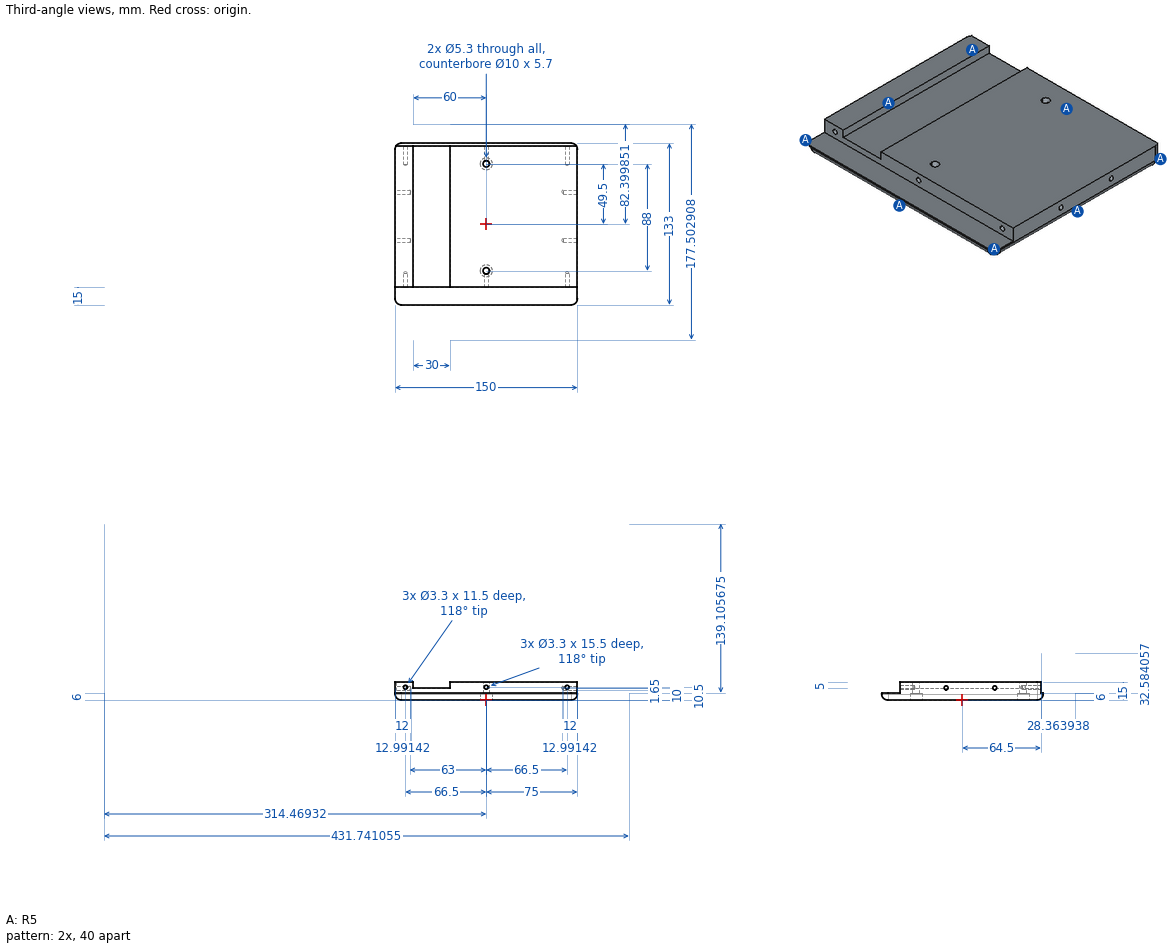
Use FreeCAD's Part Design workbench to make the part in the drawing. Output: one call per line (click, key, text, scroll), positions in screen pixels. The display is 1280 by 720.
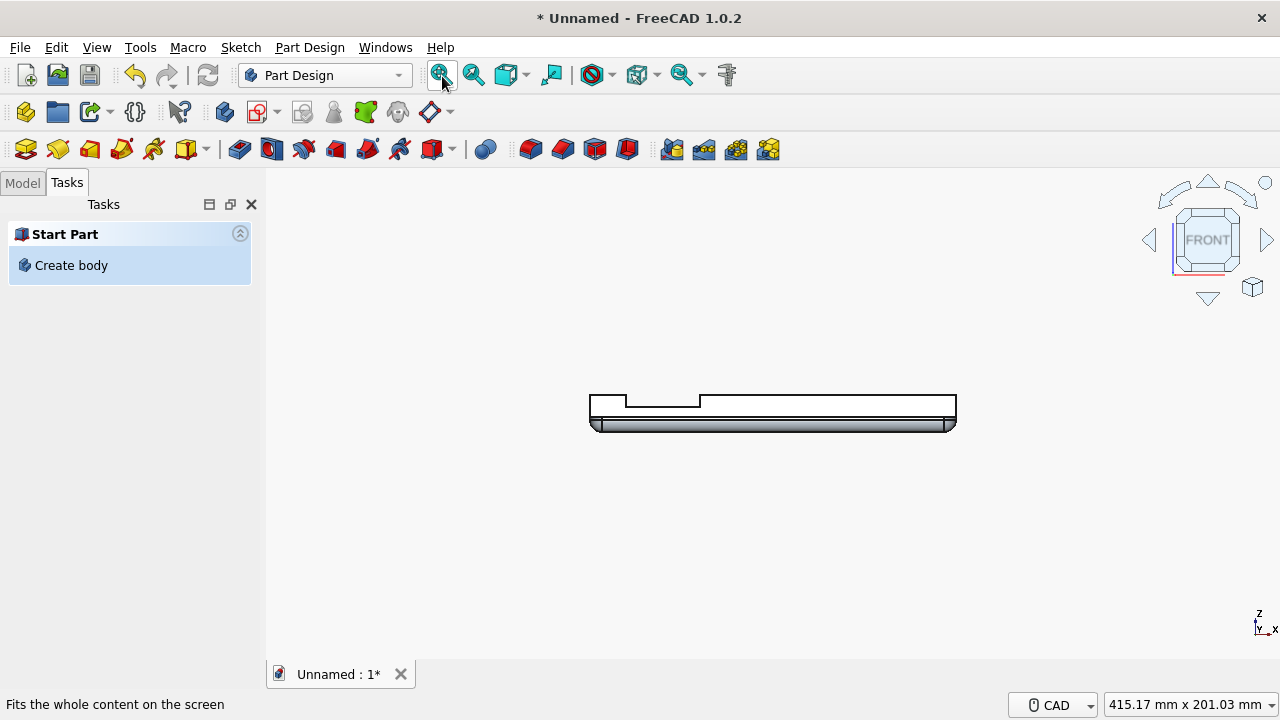
click(930, 405)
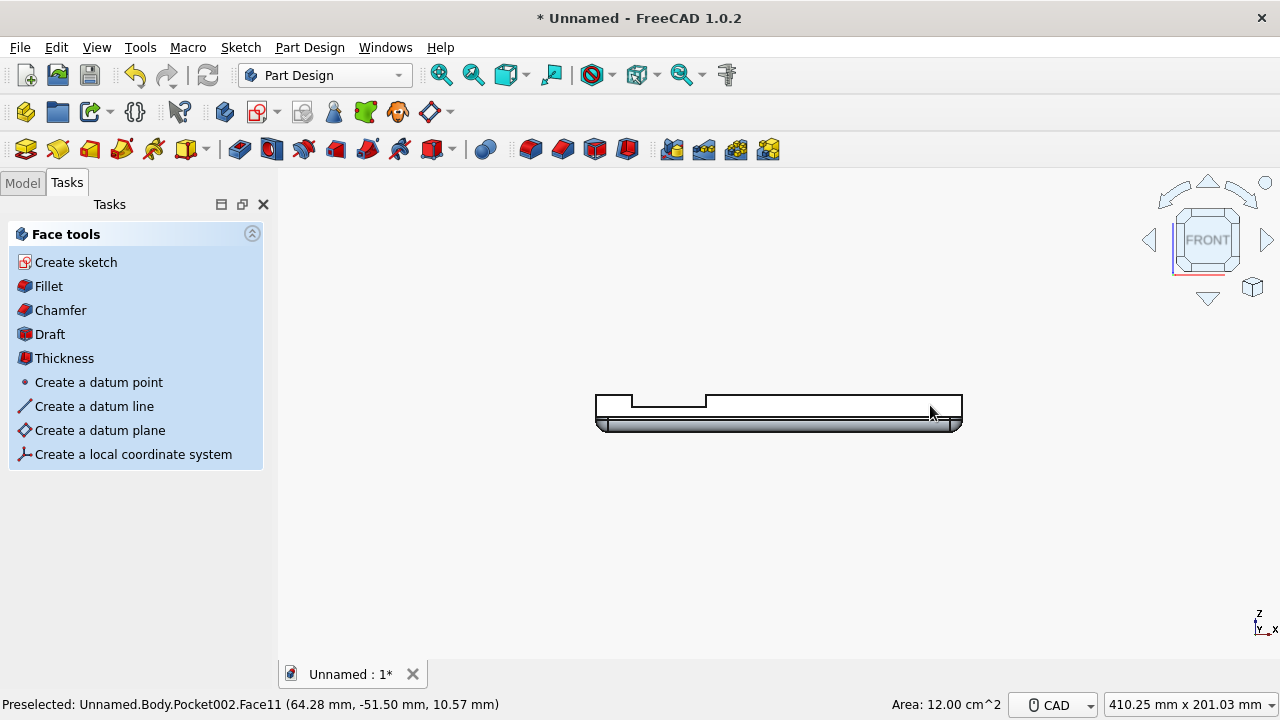
click(258, 112)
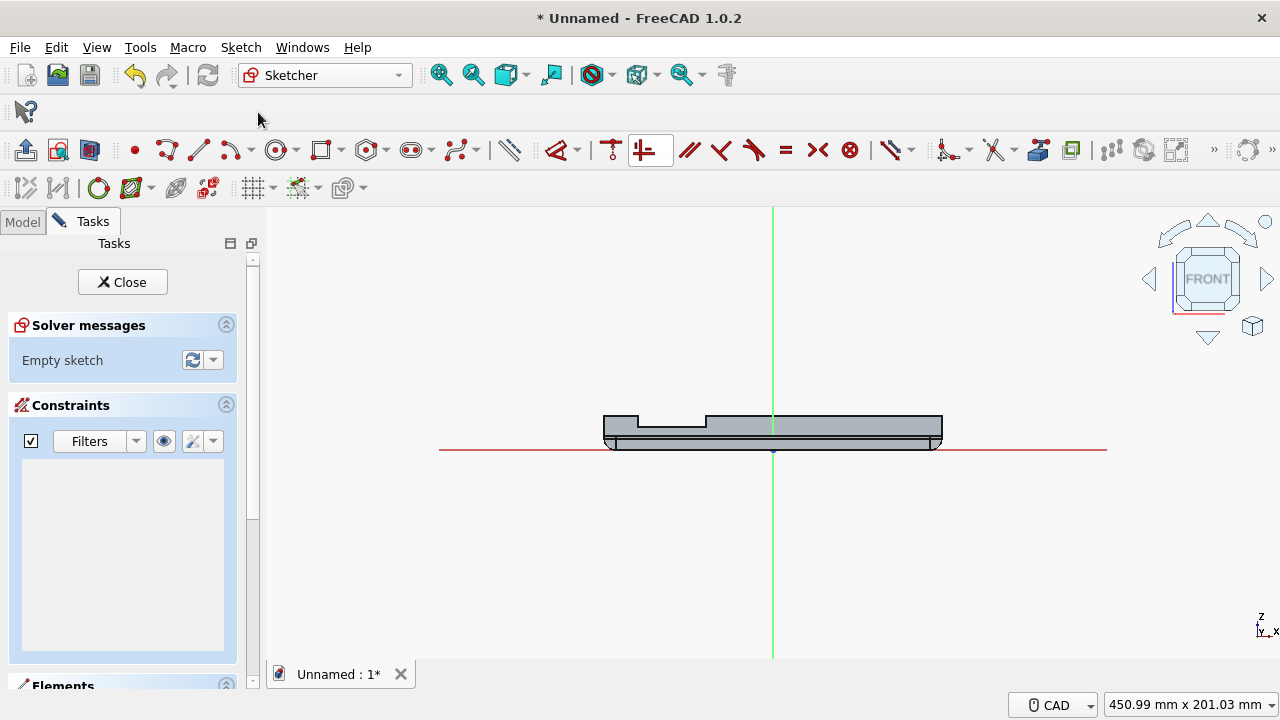
click(90, 150)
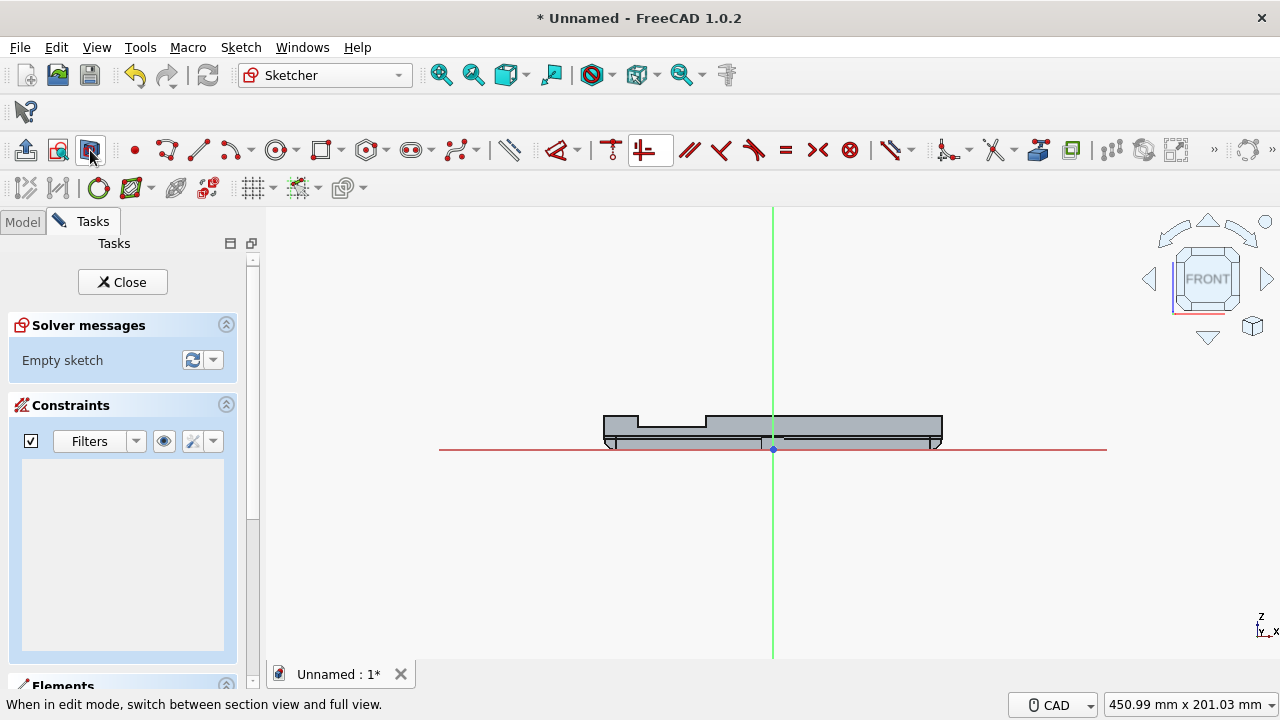
scroll(856, 440, up, 3)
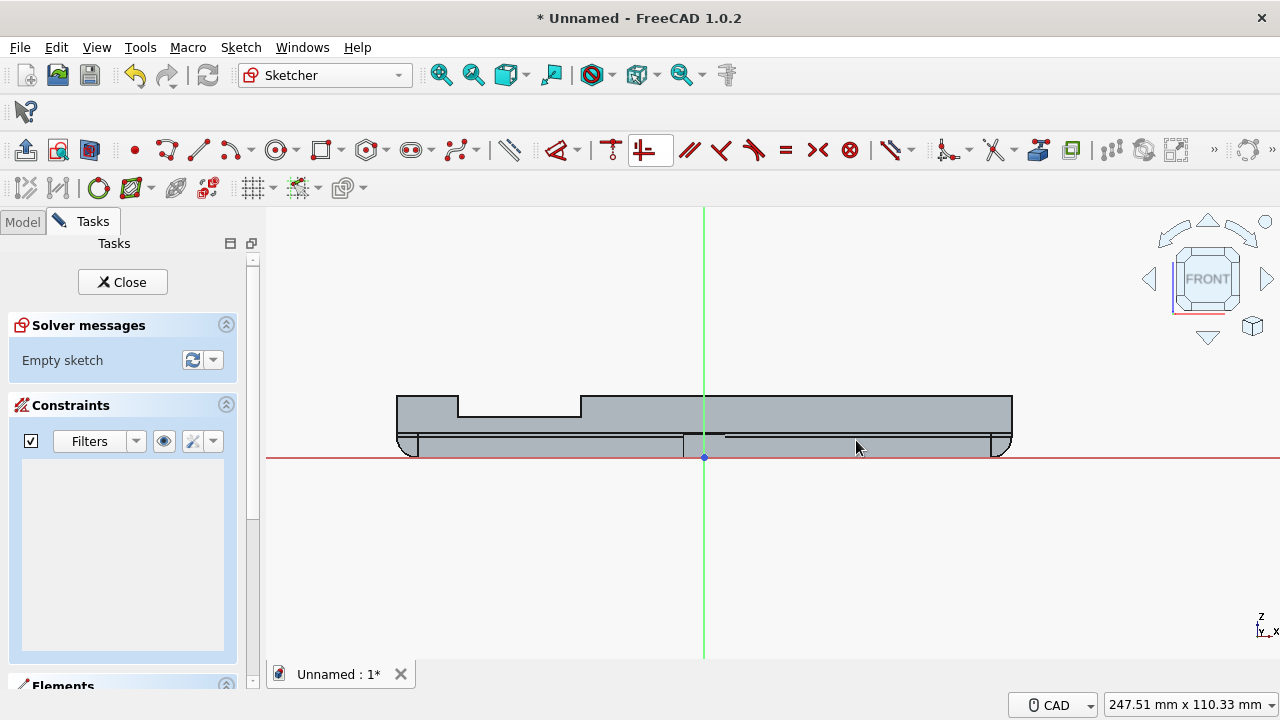
click(276, 150)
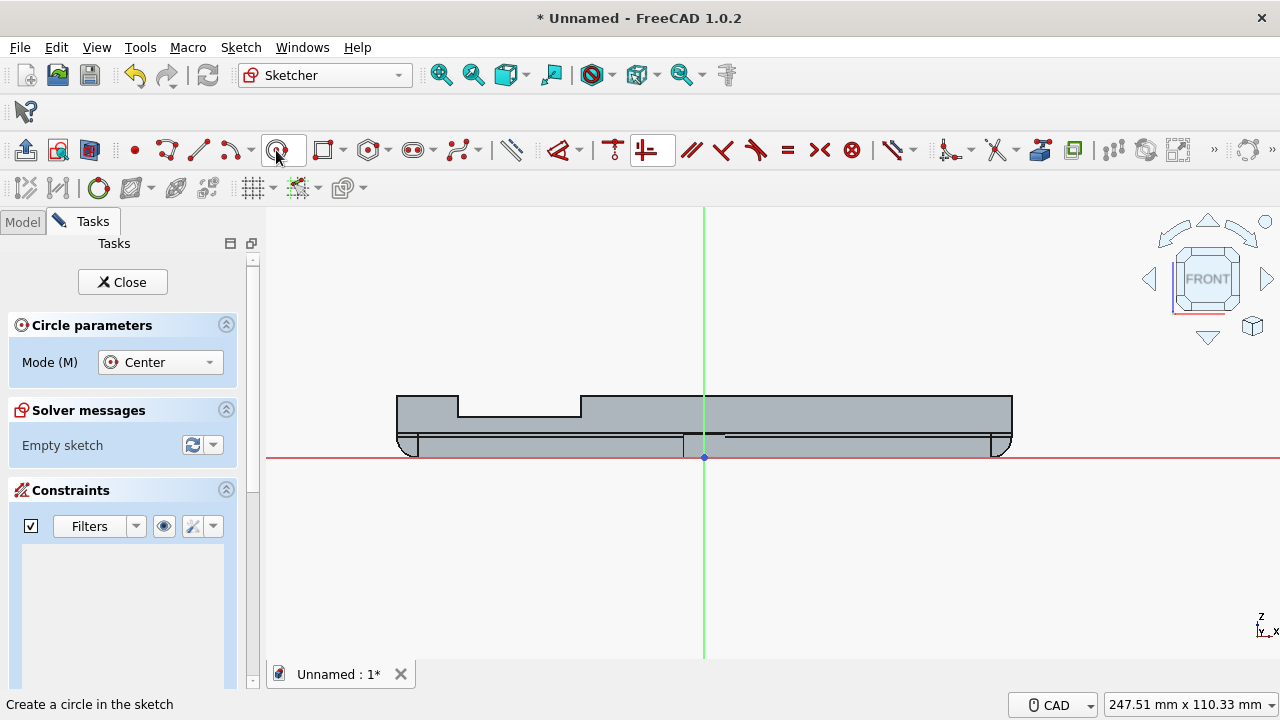
scroll(432, 415, up, 7)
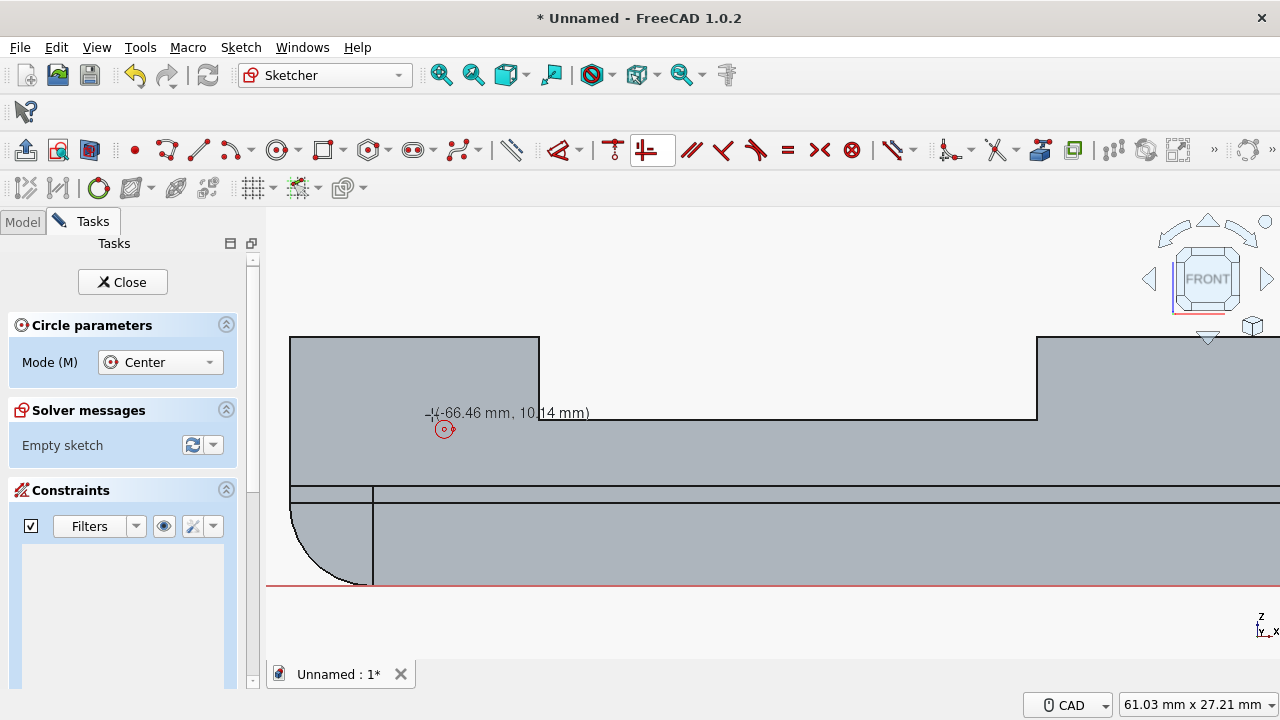
scroll(432, 416, down, 7)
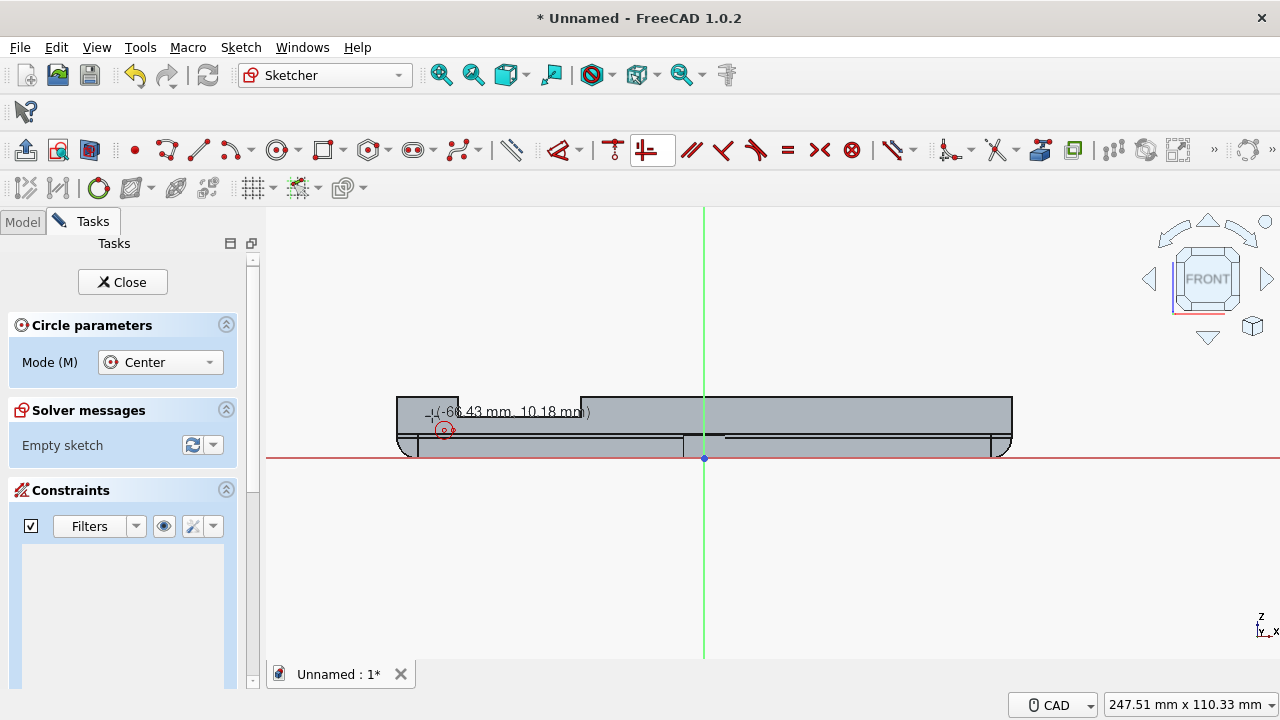
click(432, 415)
move(437, 411)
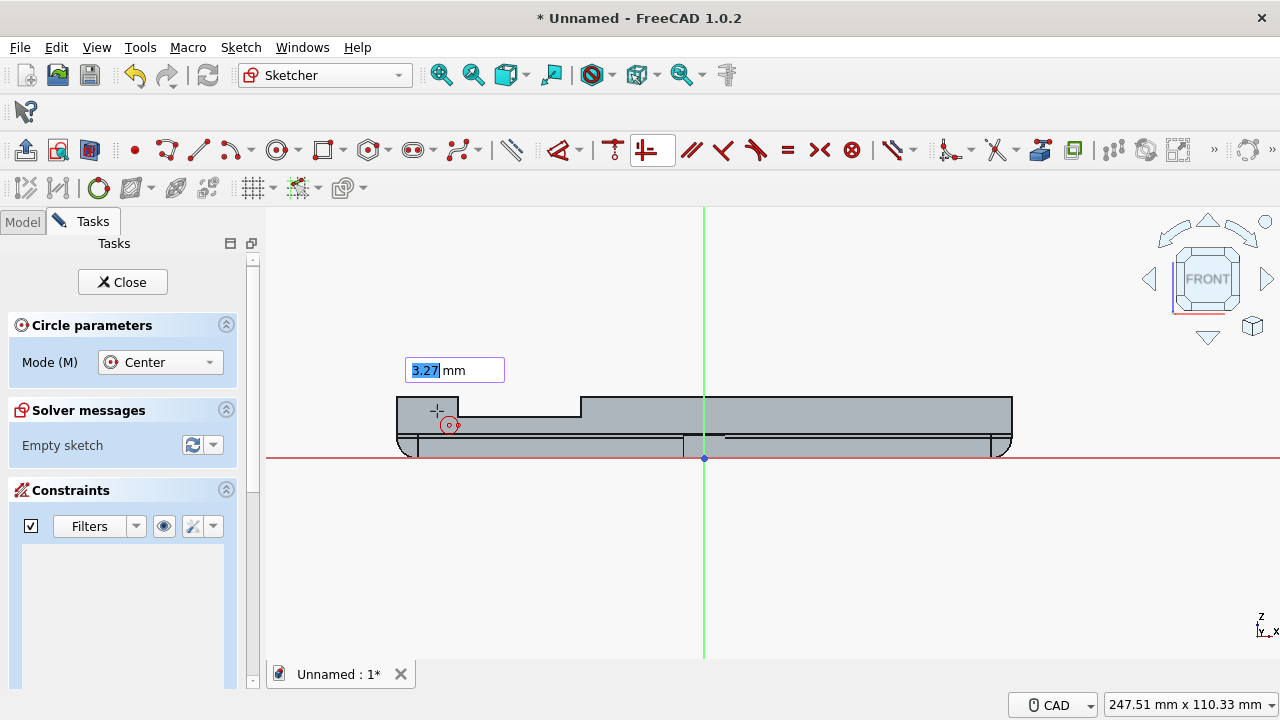
text(3.3)
key(Return)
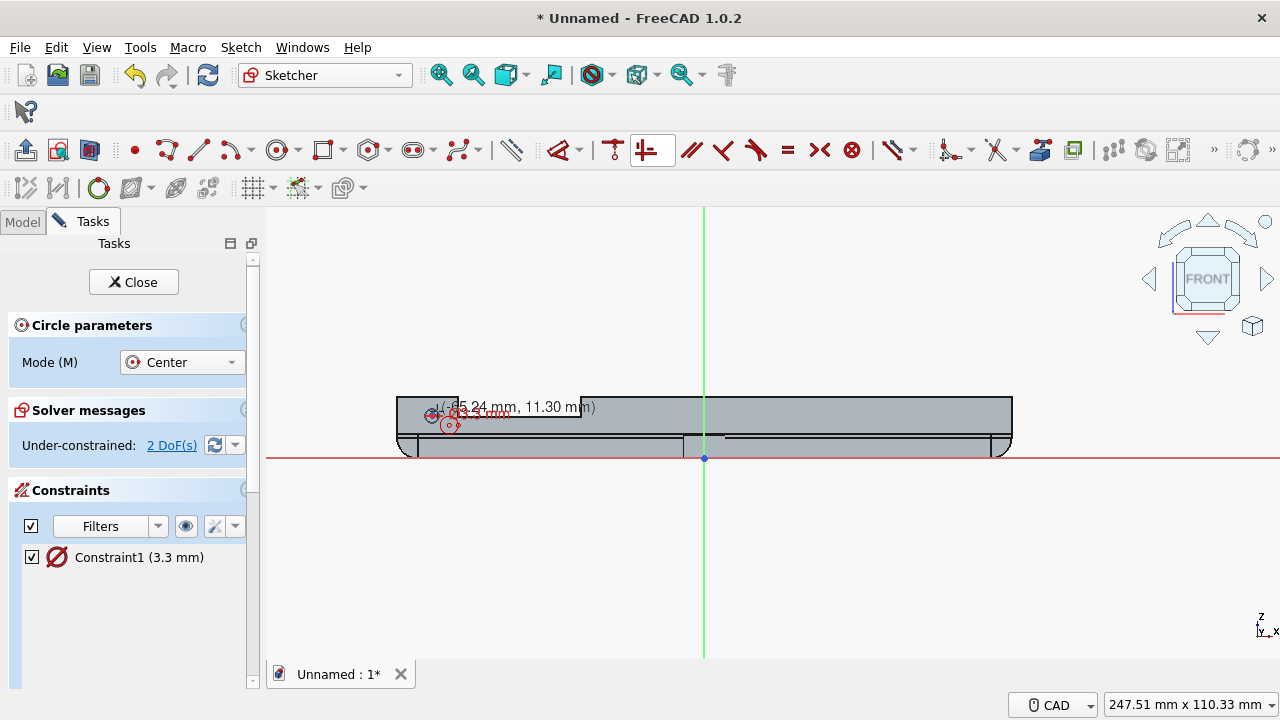
scroll(704, 415, up, 7)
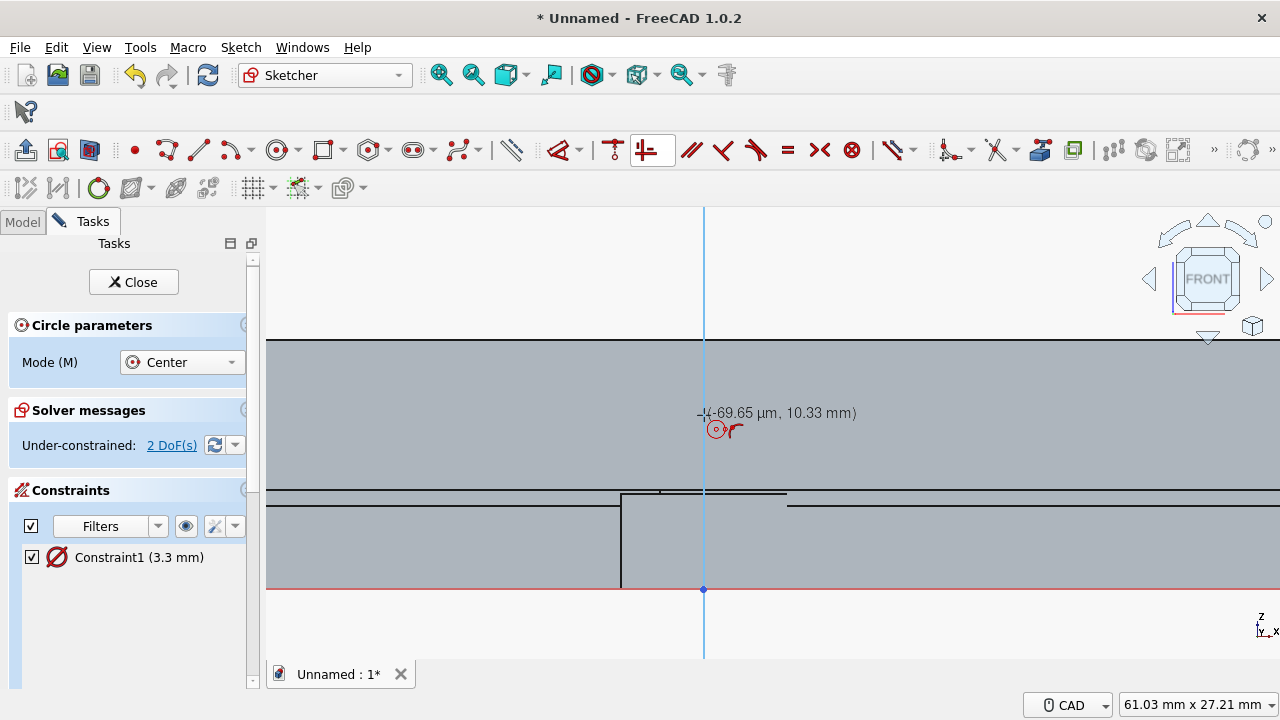
scroll(705, 415, down, 7)